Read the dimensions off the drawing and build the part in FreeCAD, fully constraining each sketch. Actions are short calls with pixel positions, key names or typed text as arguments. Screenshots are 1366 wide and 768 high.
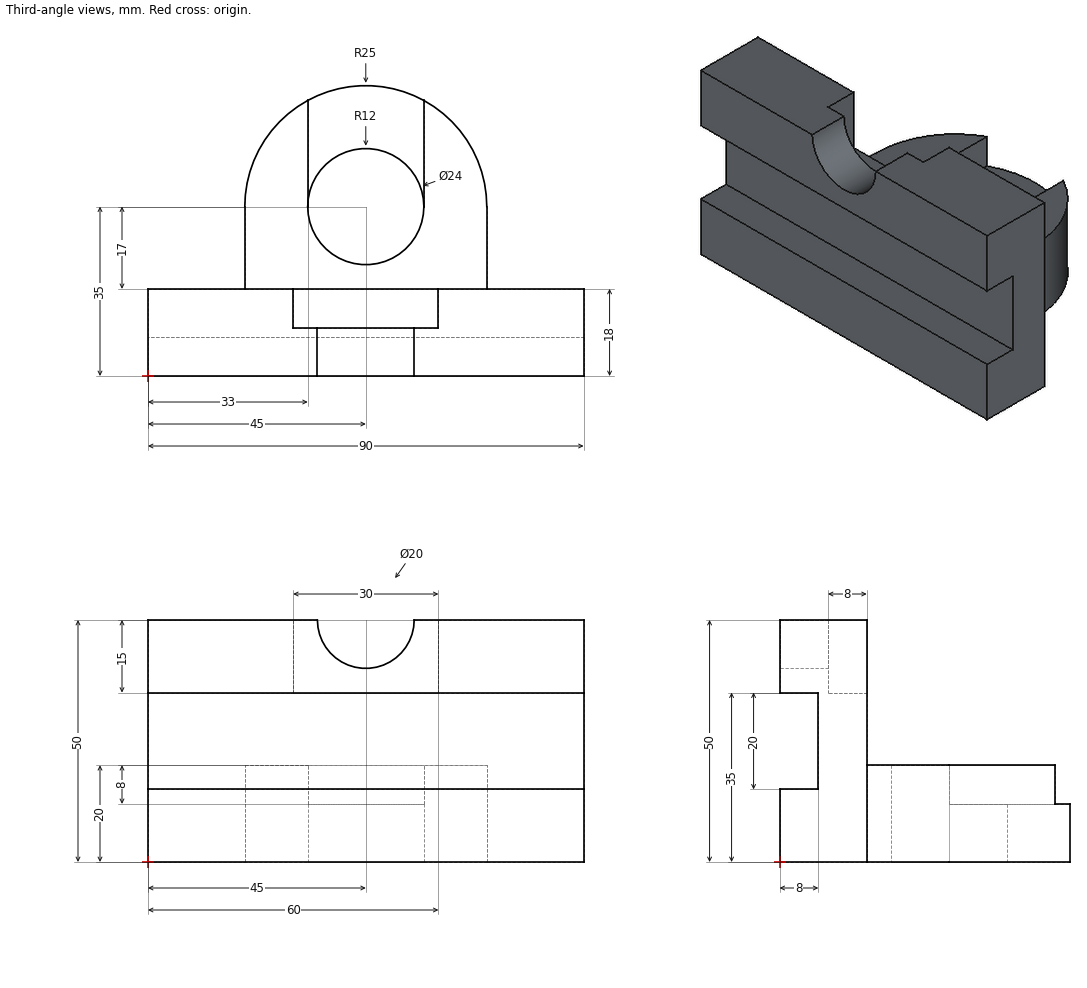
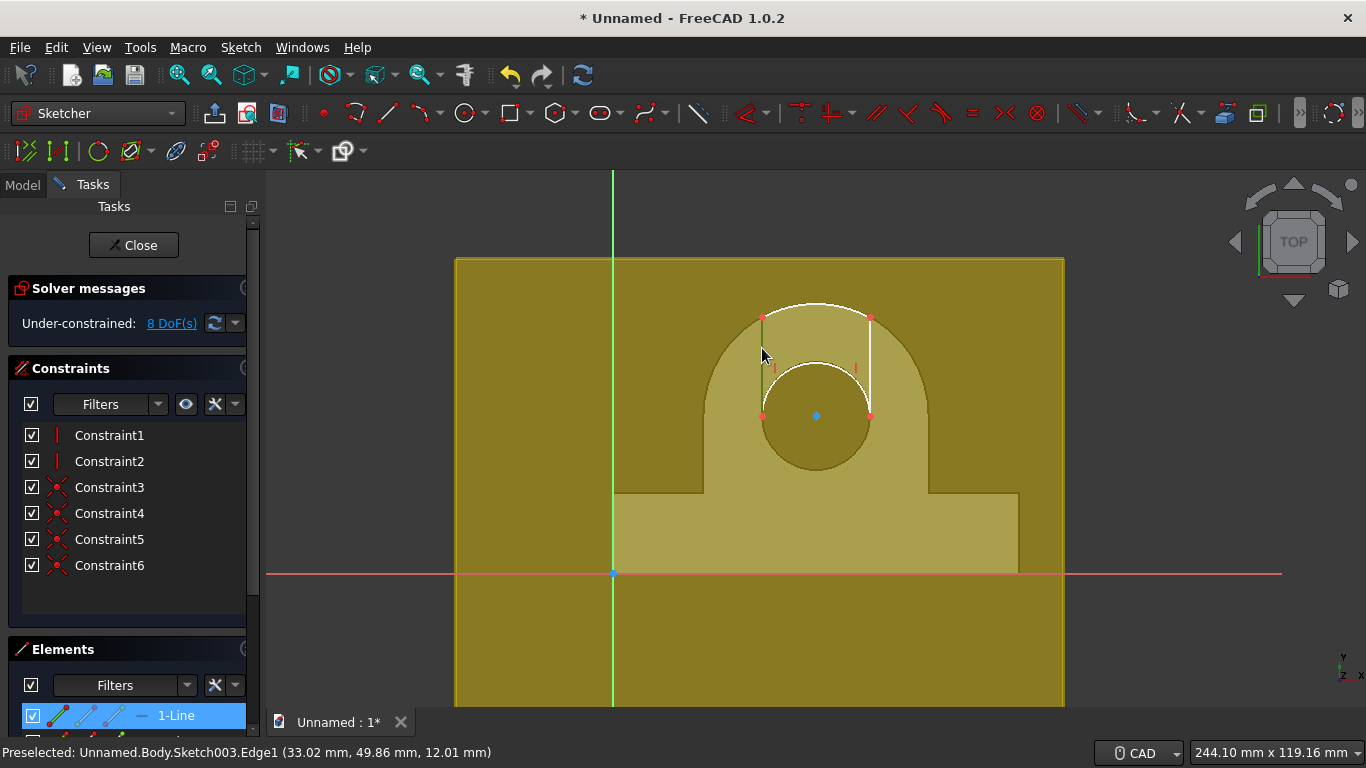
click(848, 373)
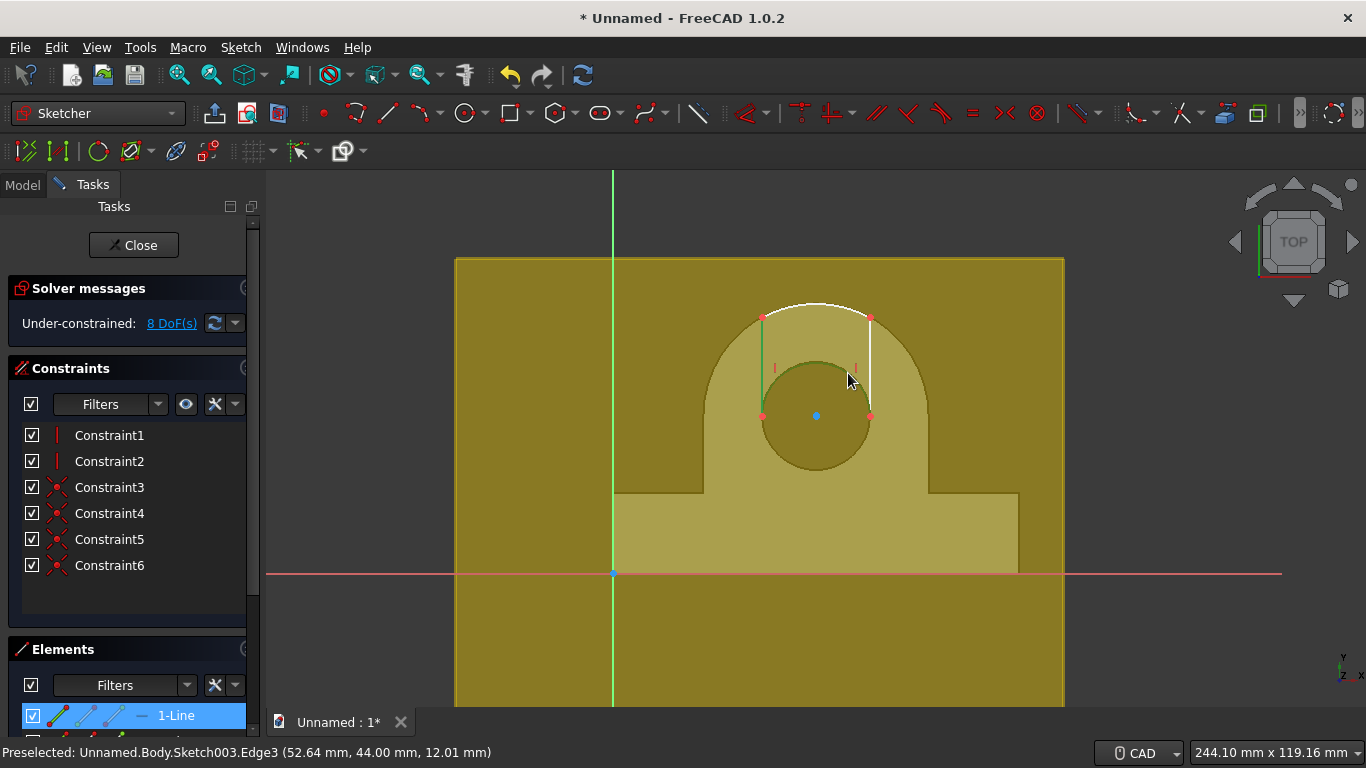
click(942, 114)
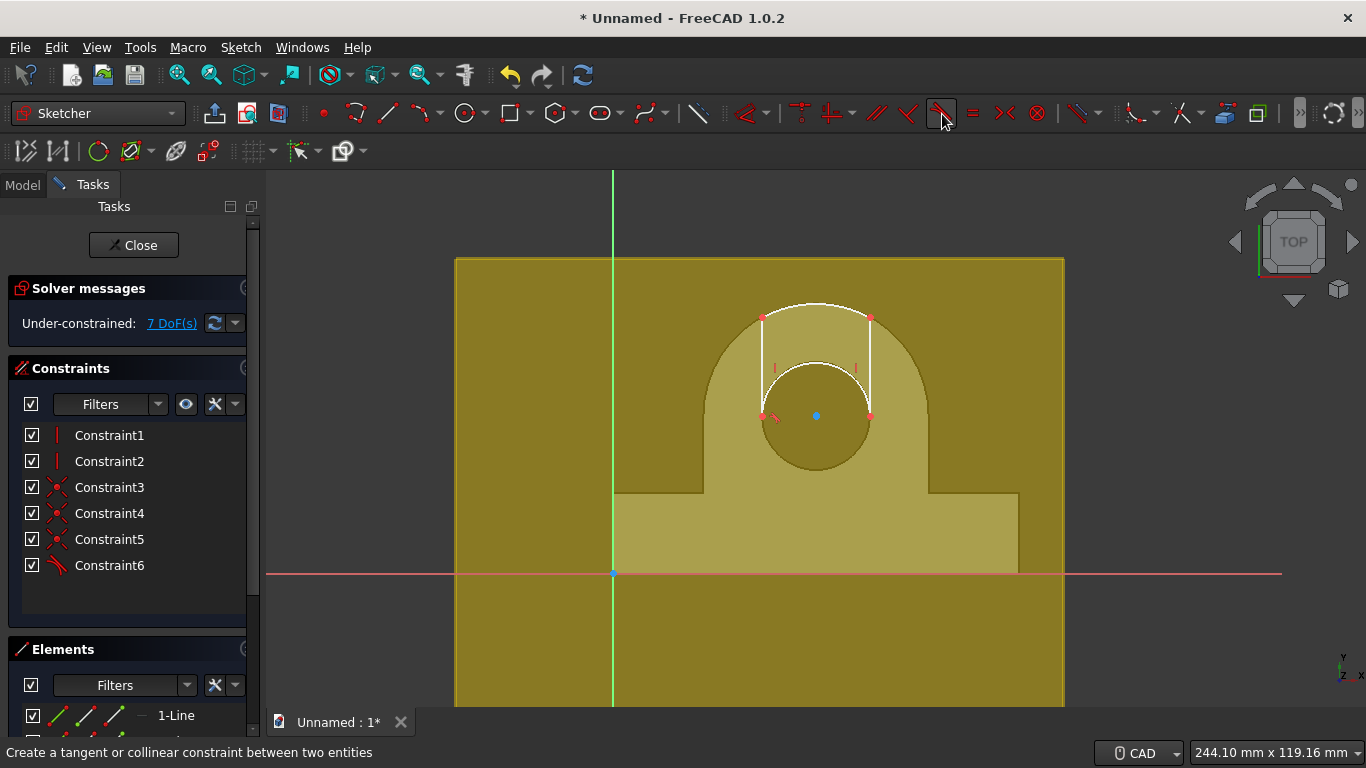
click(870, 348)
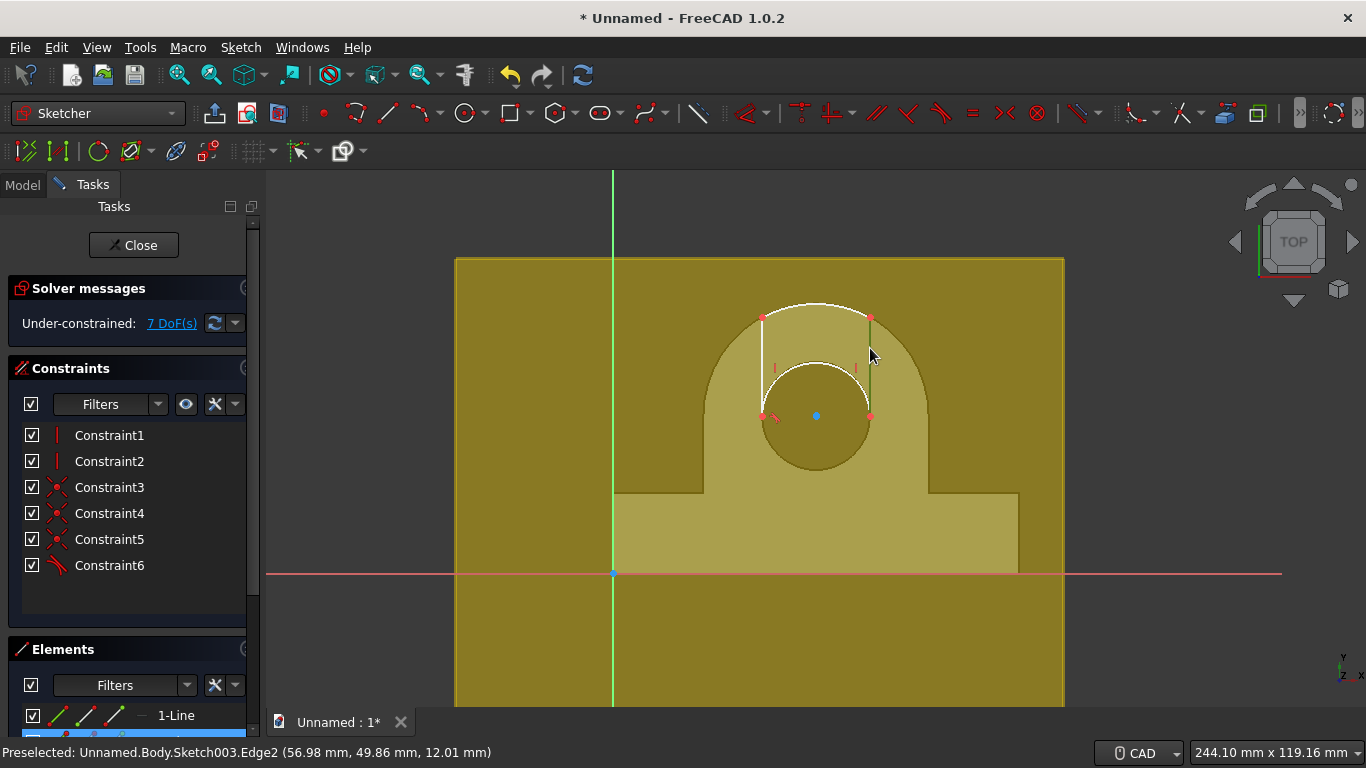
click(848, 373)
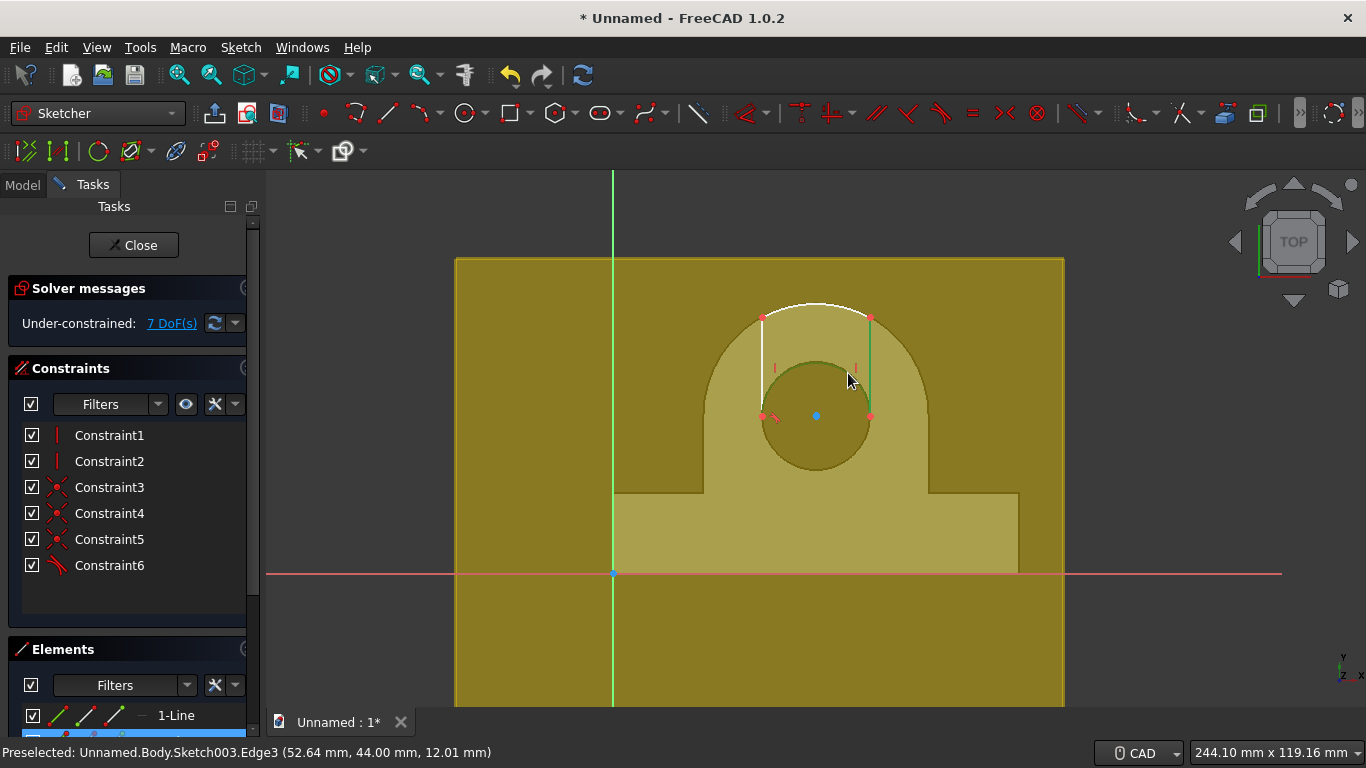
click(942, 114)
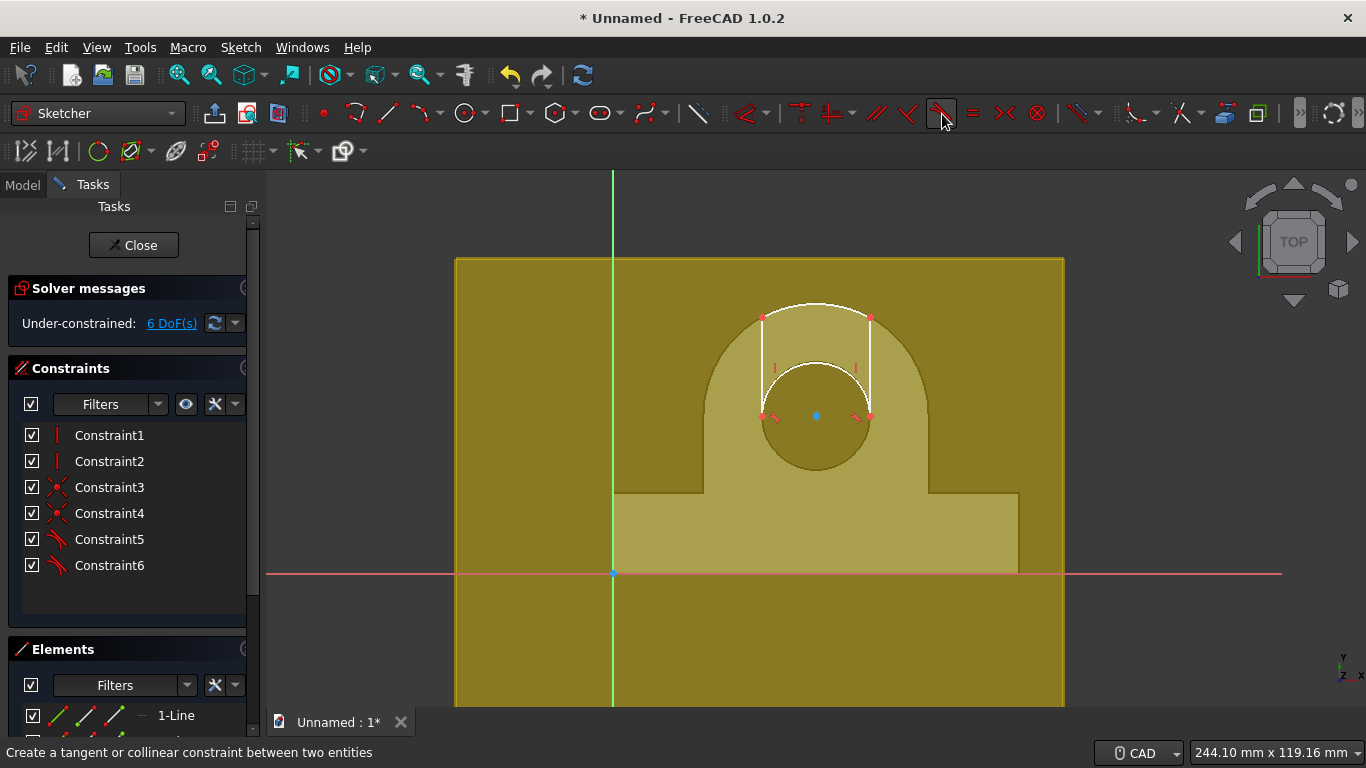
click(848, 373)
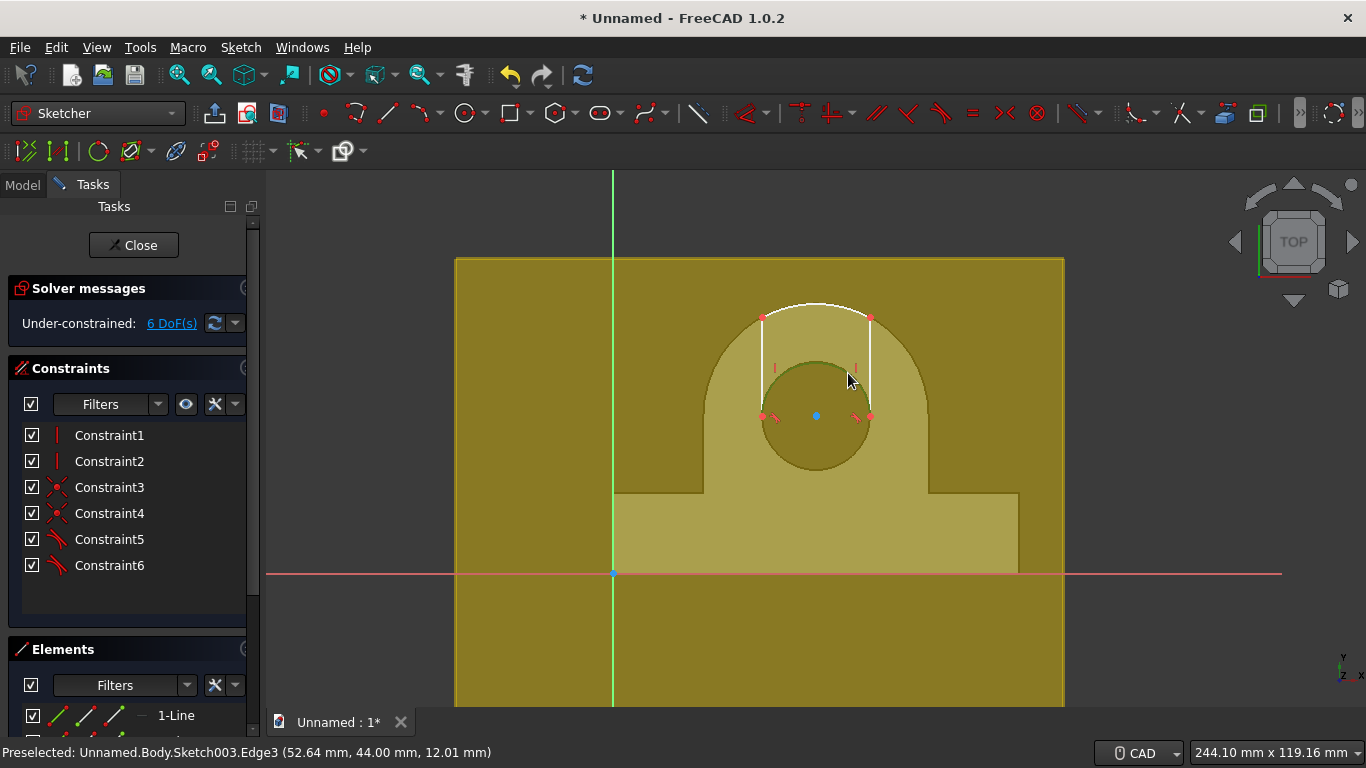
click(838, 306)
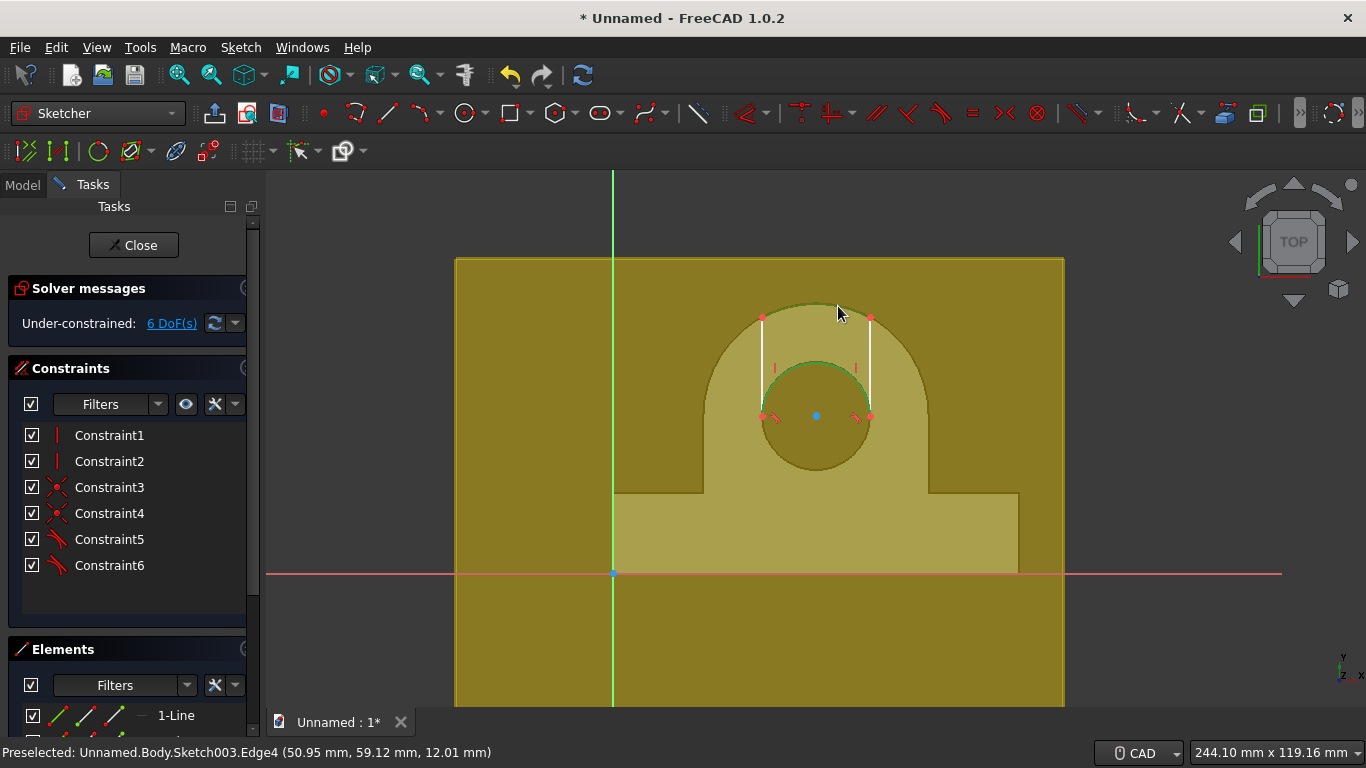
key(c)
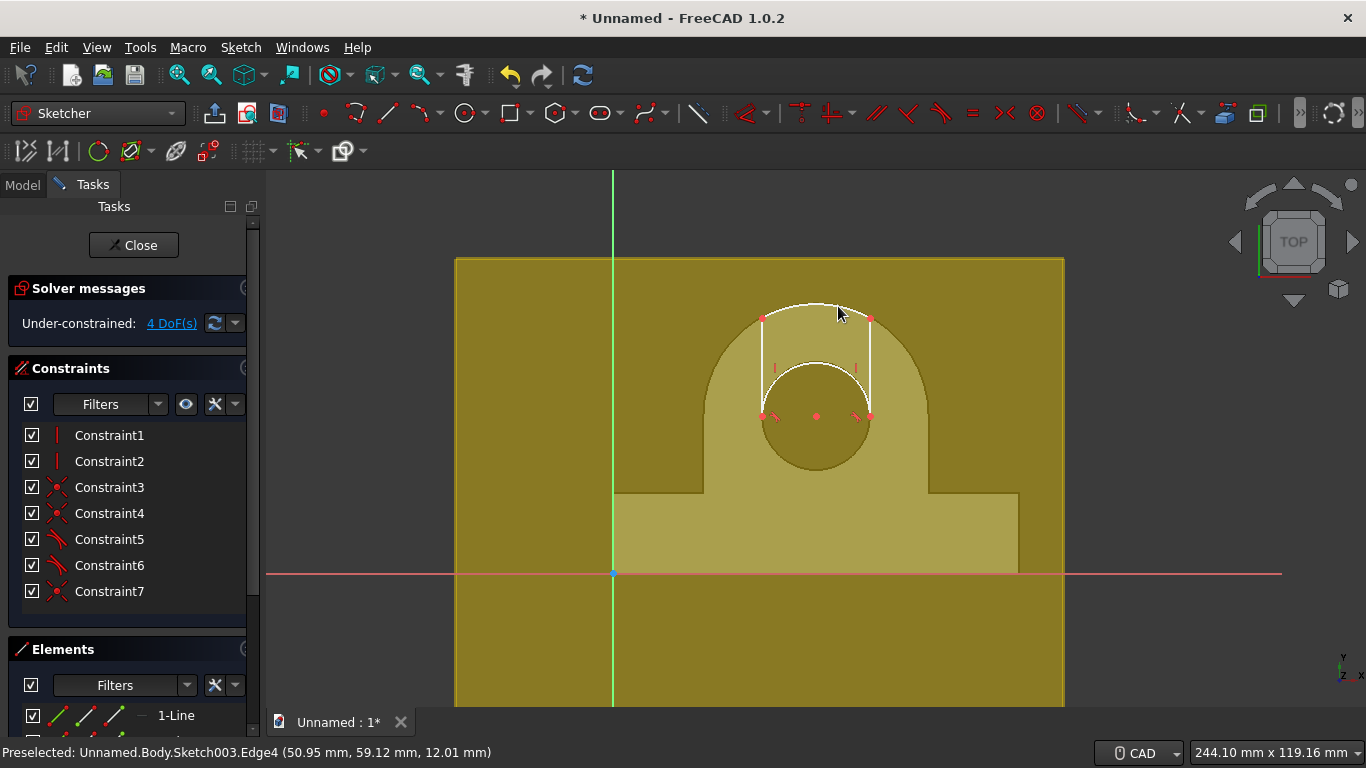
key(d)